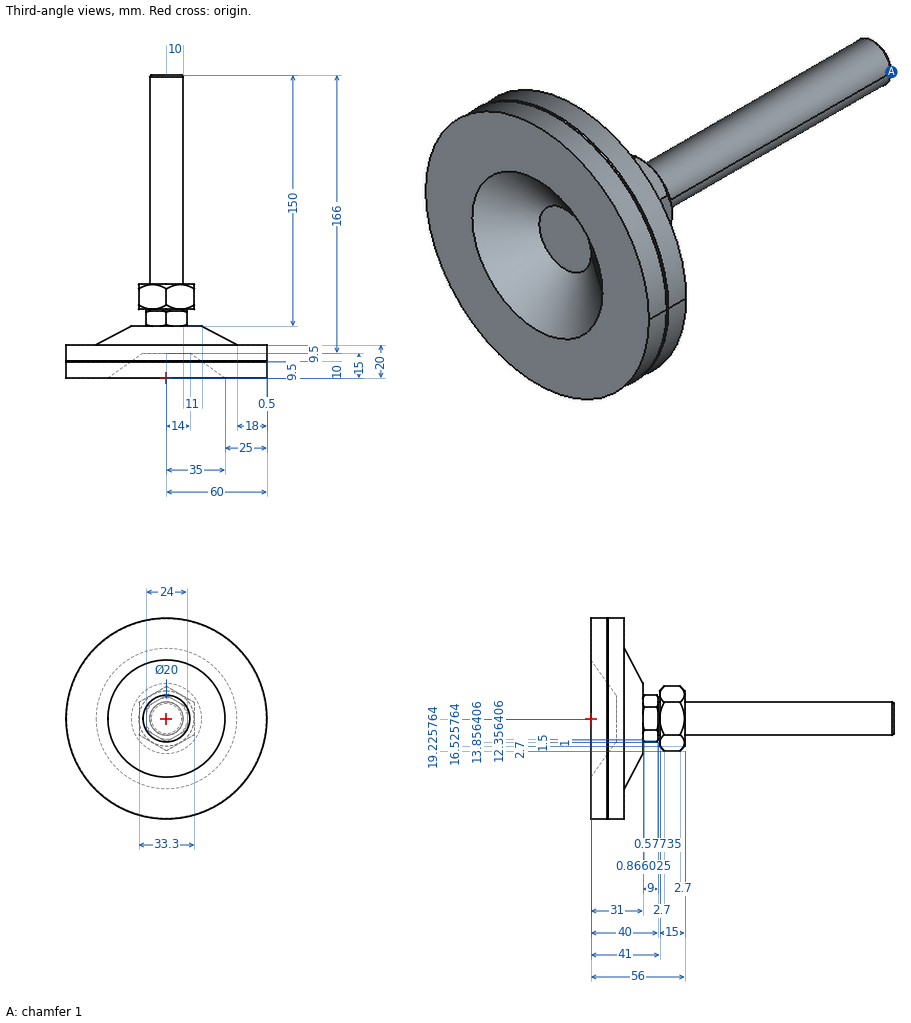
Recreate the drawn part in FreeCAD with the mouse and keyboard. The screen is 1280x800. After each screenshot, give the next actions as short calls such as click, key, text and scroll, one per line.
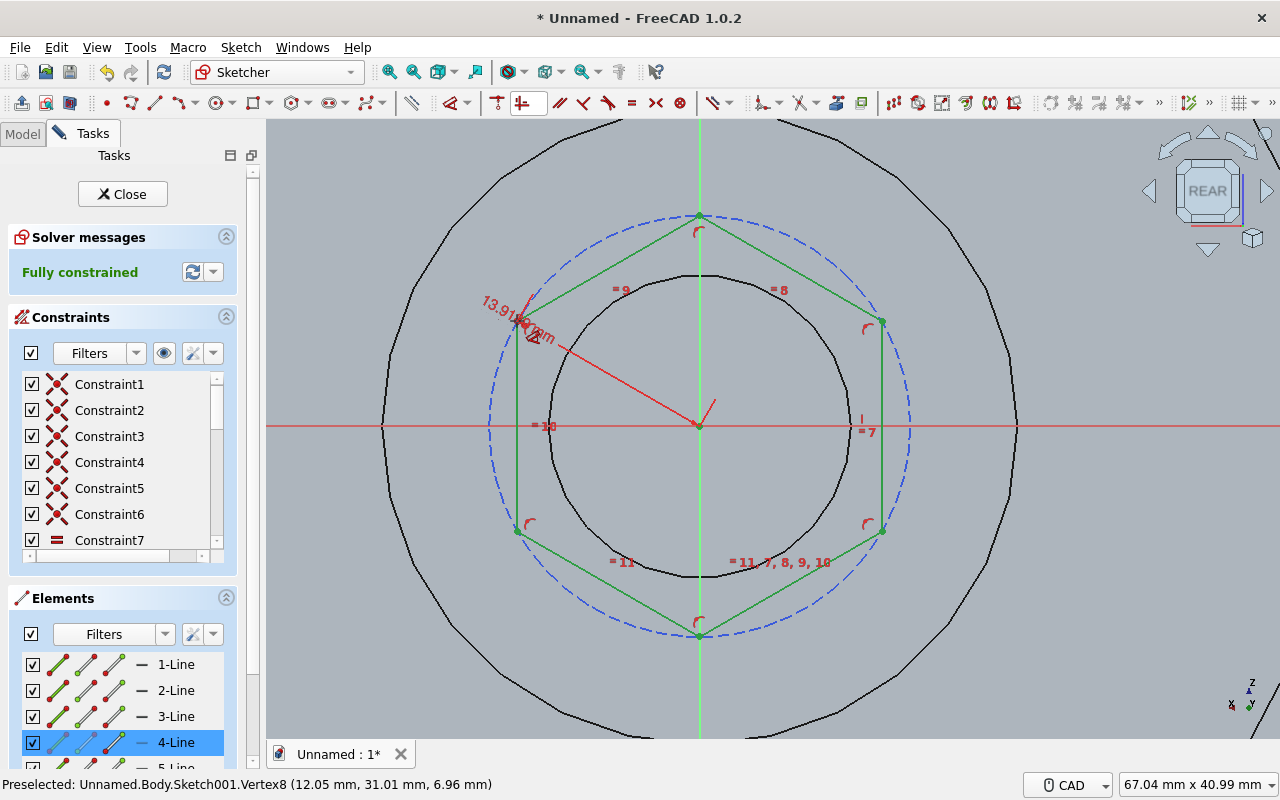
click(882, 532)
click(616, 566)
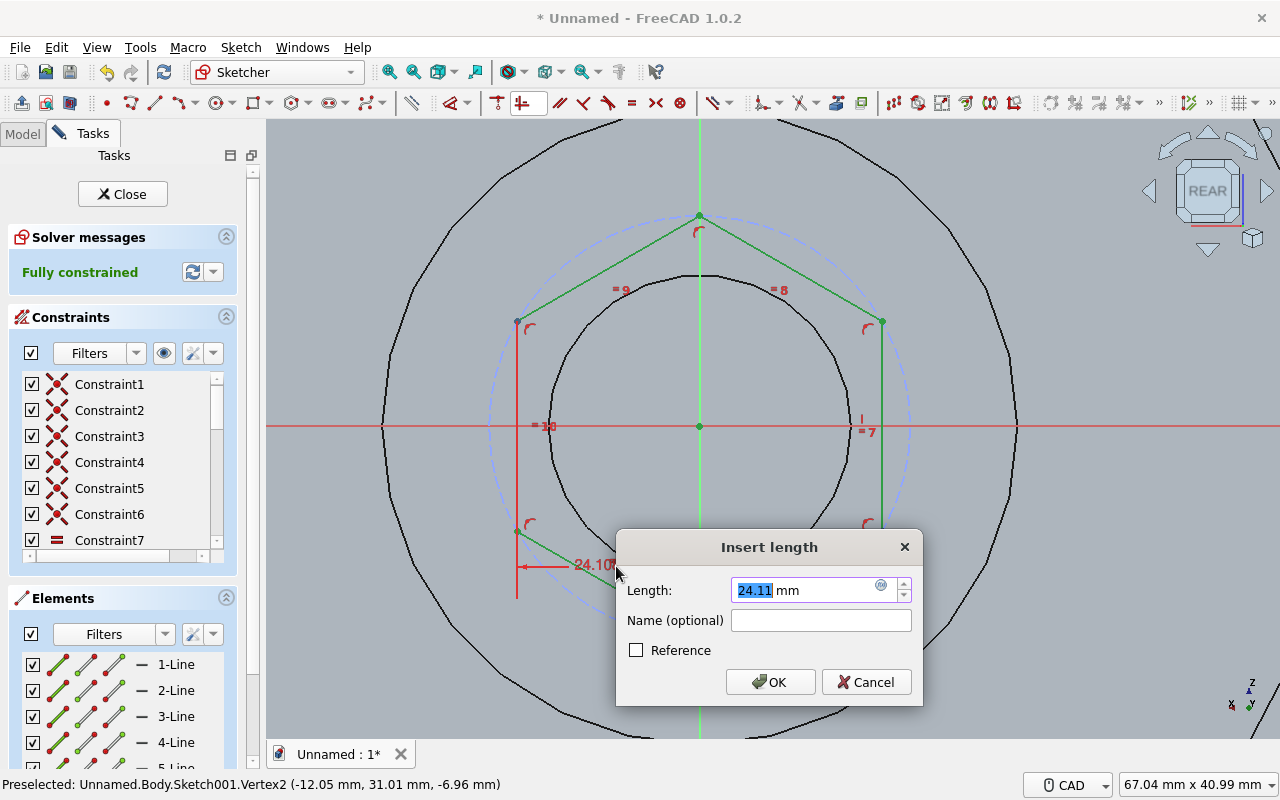
text(24)
key(Return)
key(Escape)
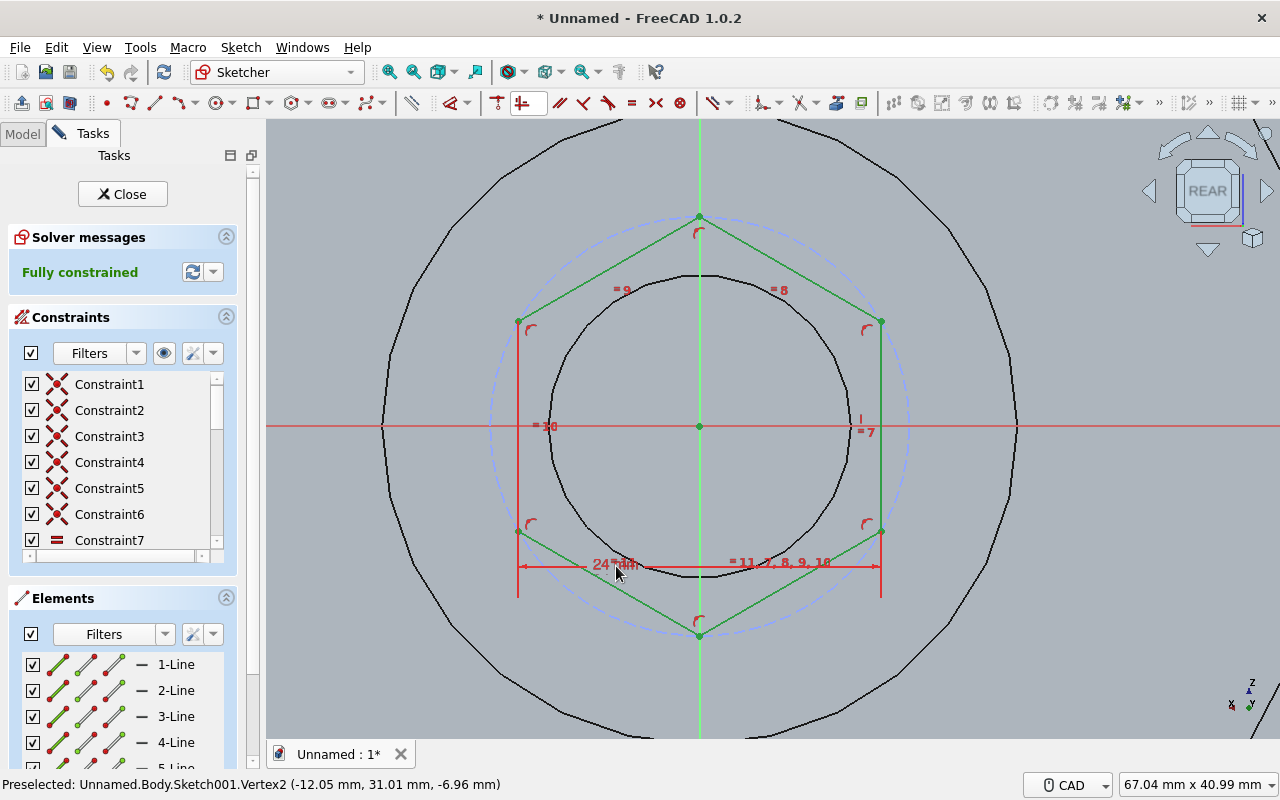
click(123, 194)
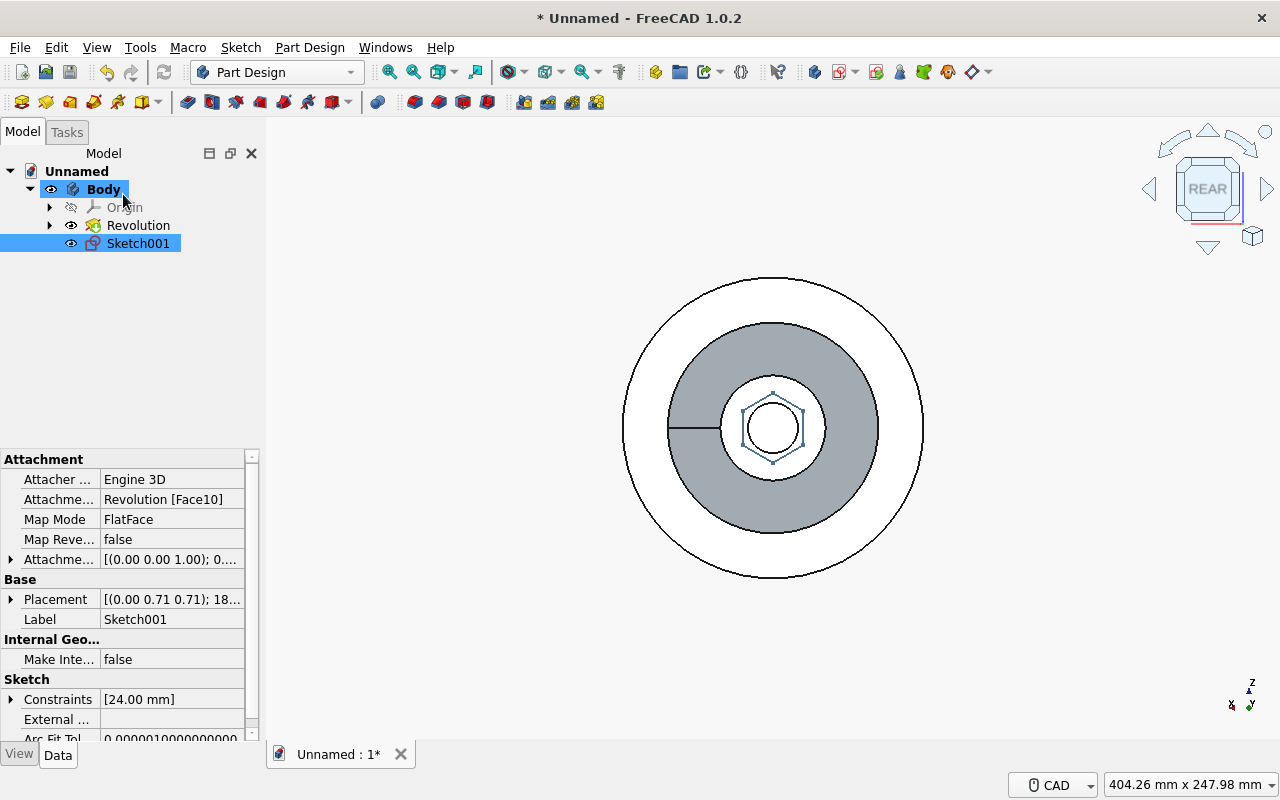
click(22, 102)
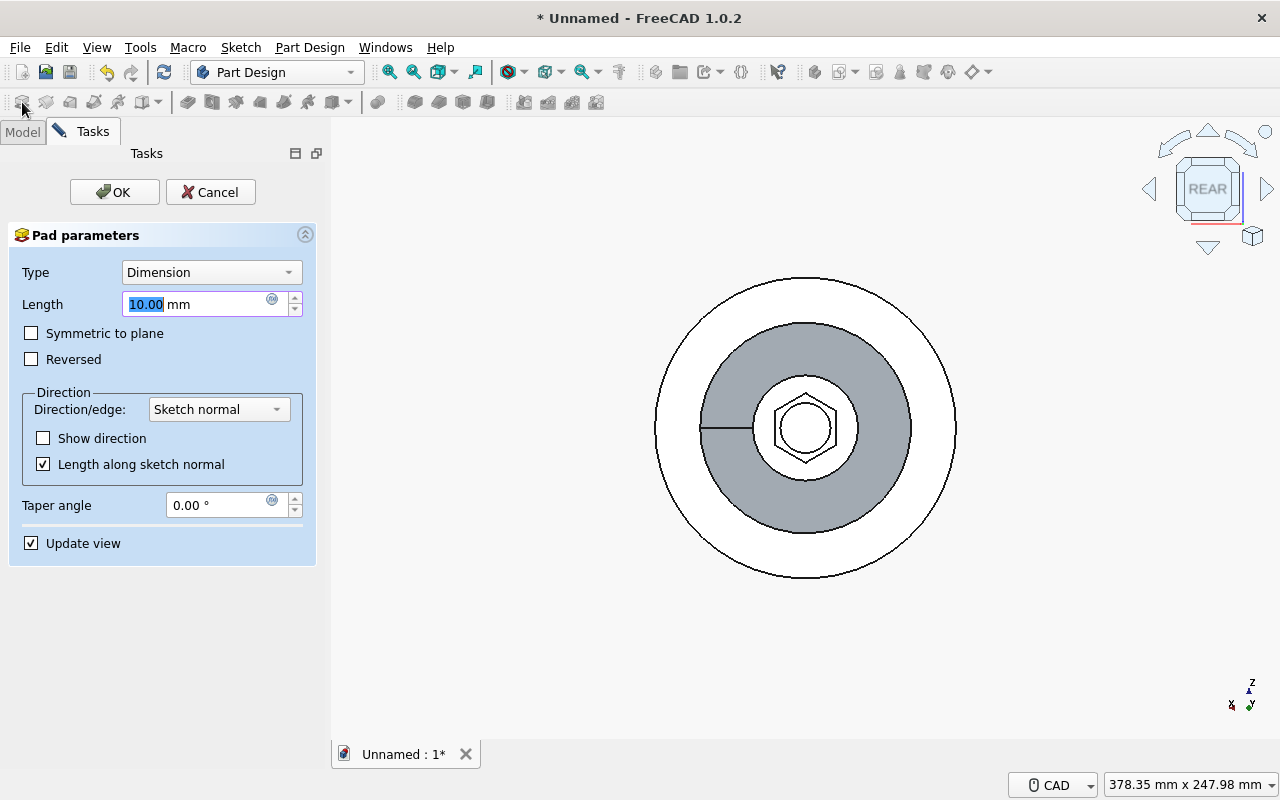
text(9)
key(Tab)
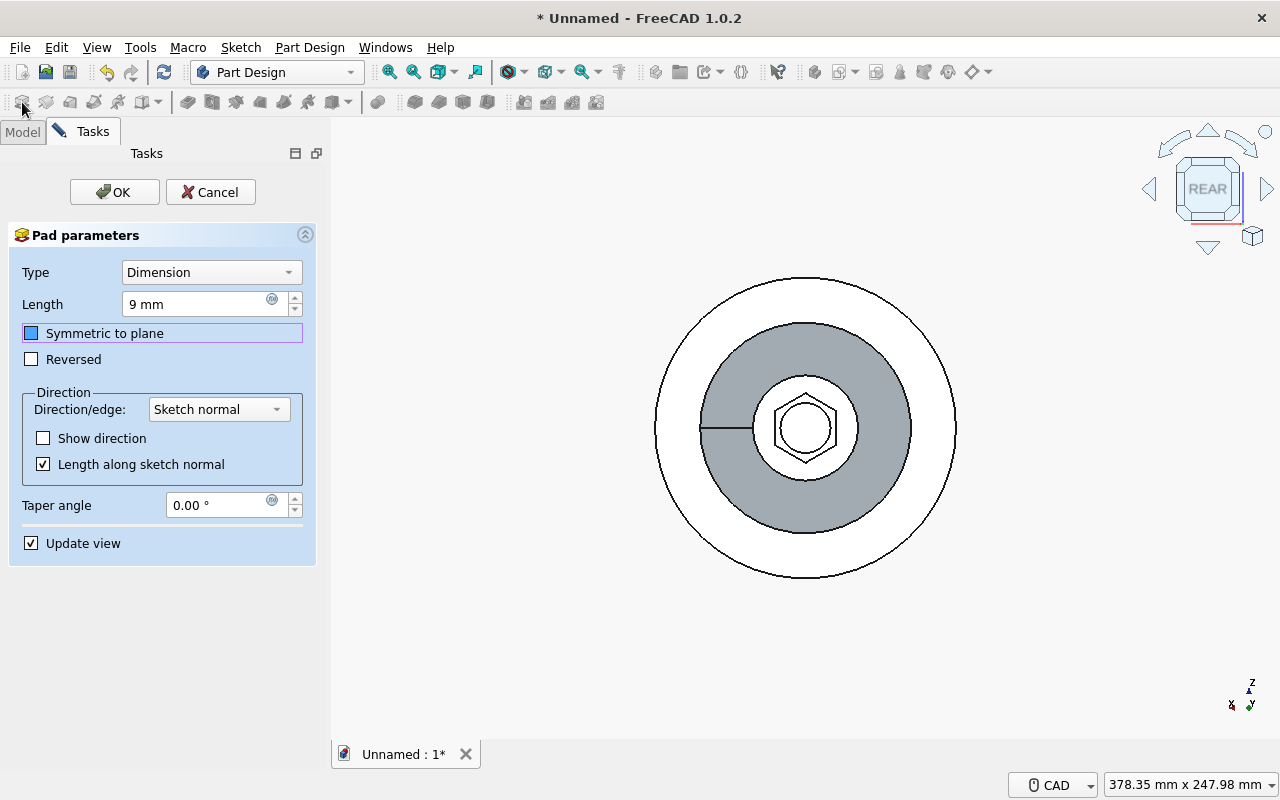
click(115, 192)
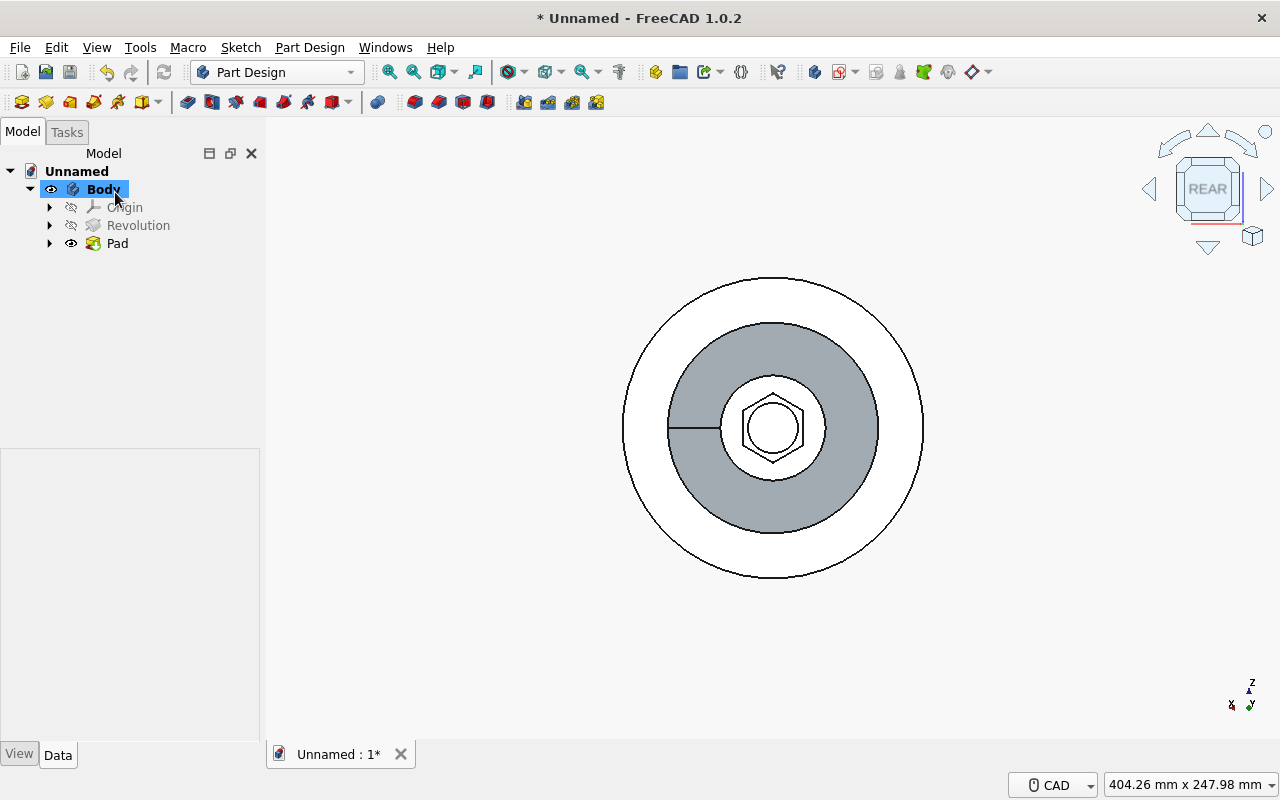
click(840, 72)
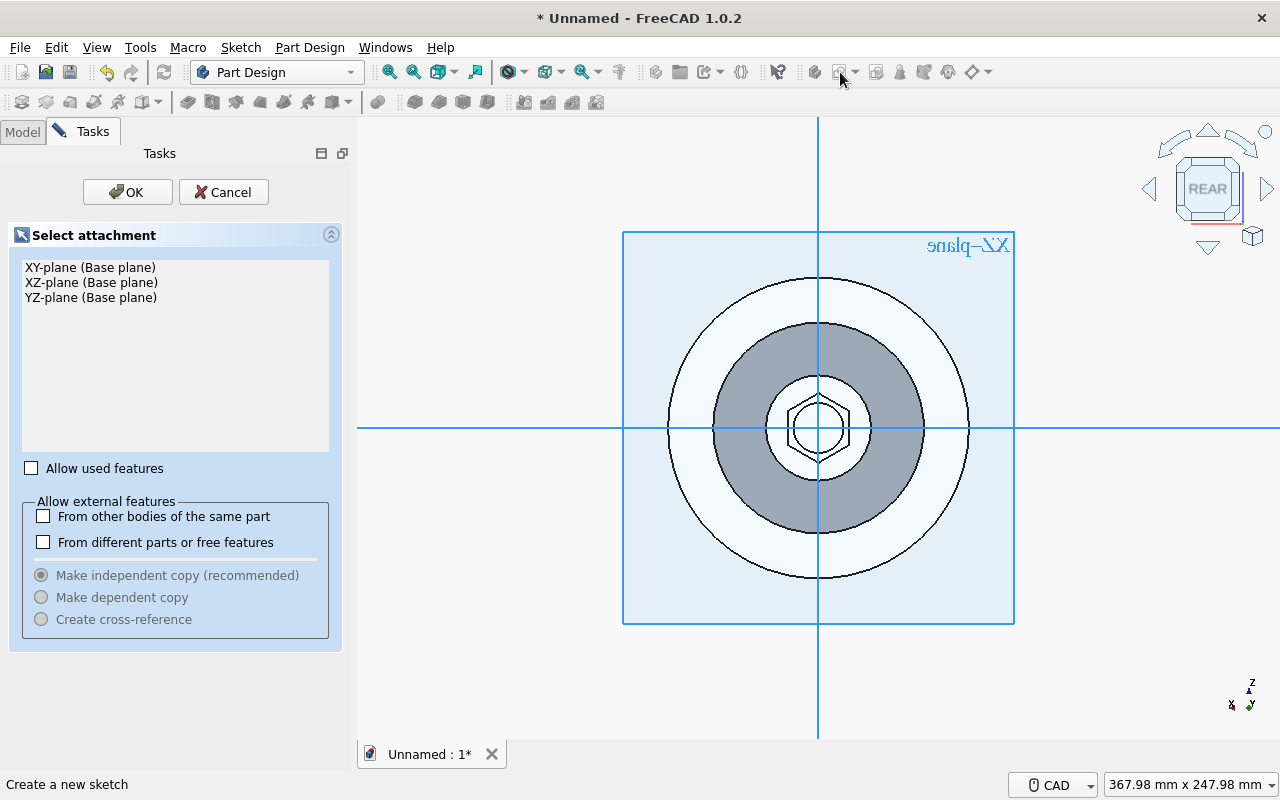
click(82, 298)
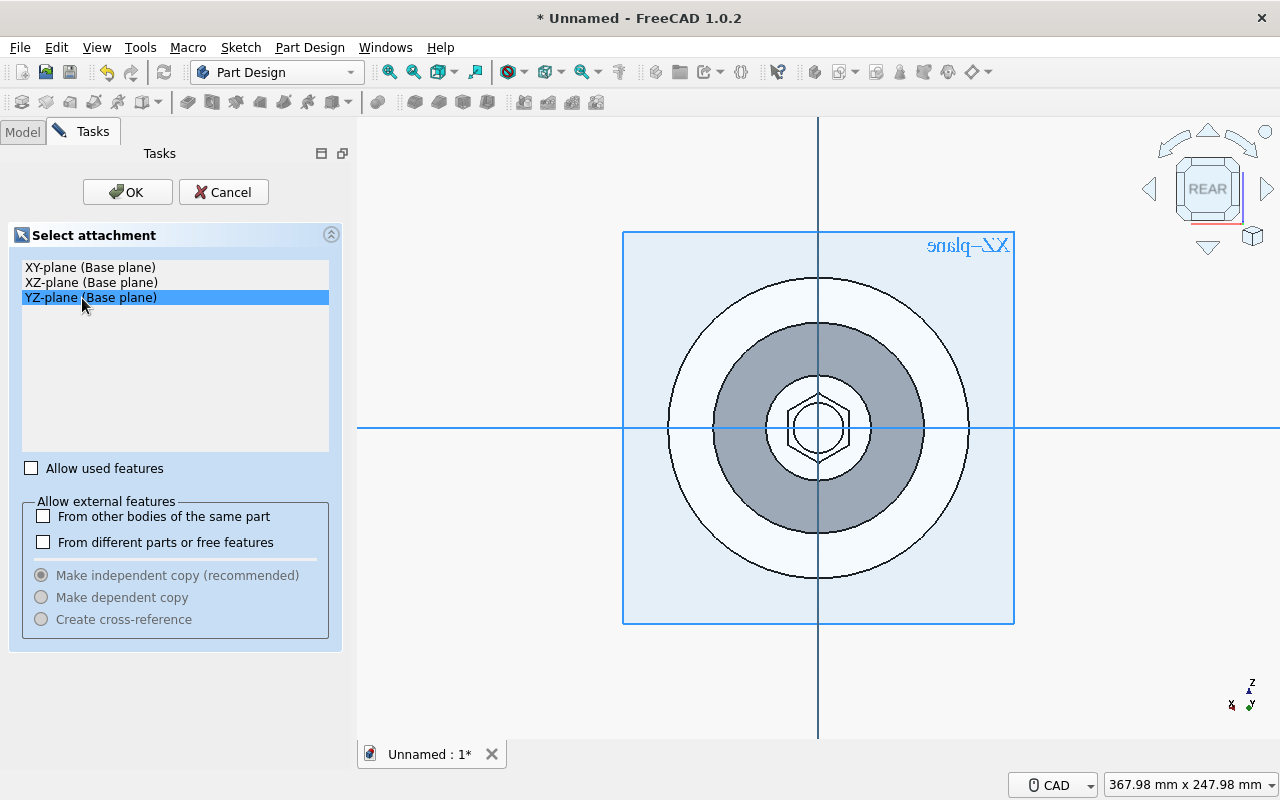
click(128, 192)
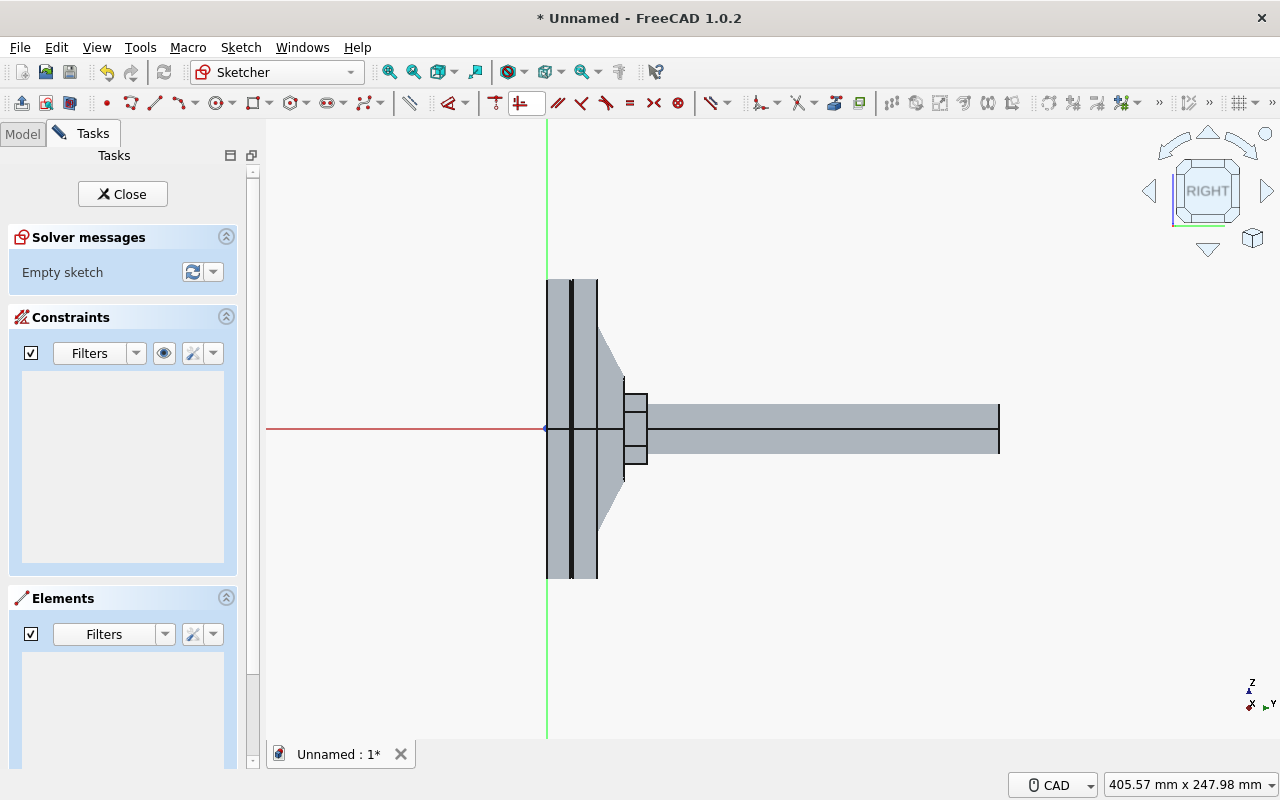
click(70, 104)